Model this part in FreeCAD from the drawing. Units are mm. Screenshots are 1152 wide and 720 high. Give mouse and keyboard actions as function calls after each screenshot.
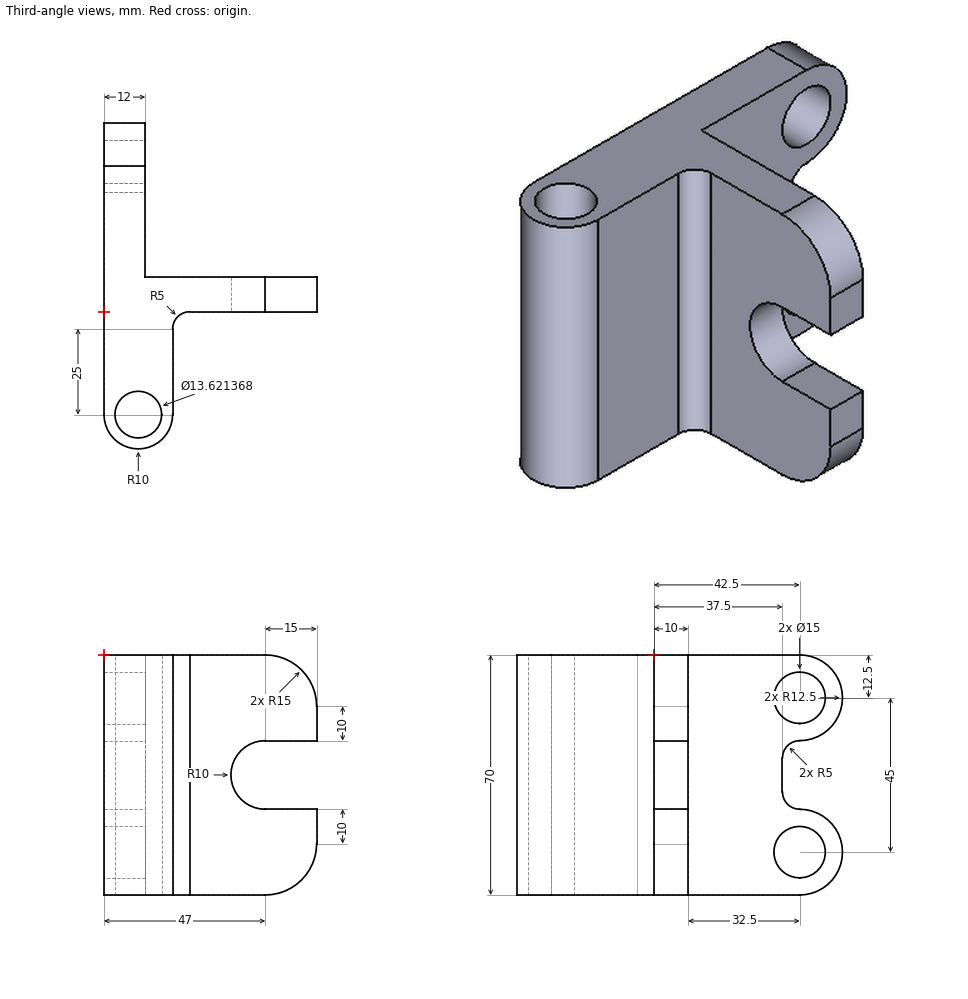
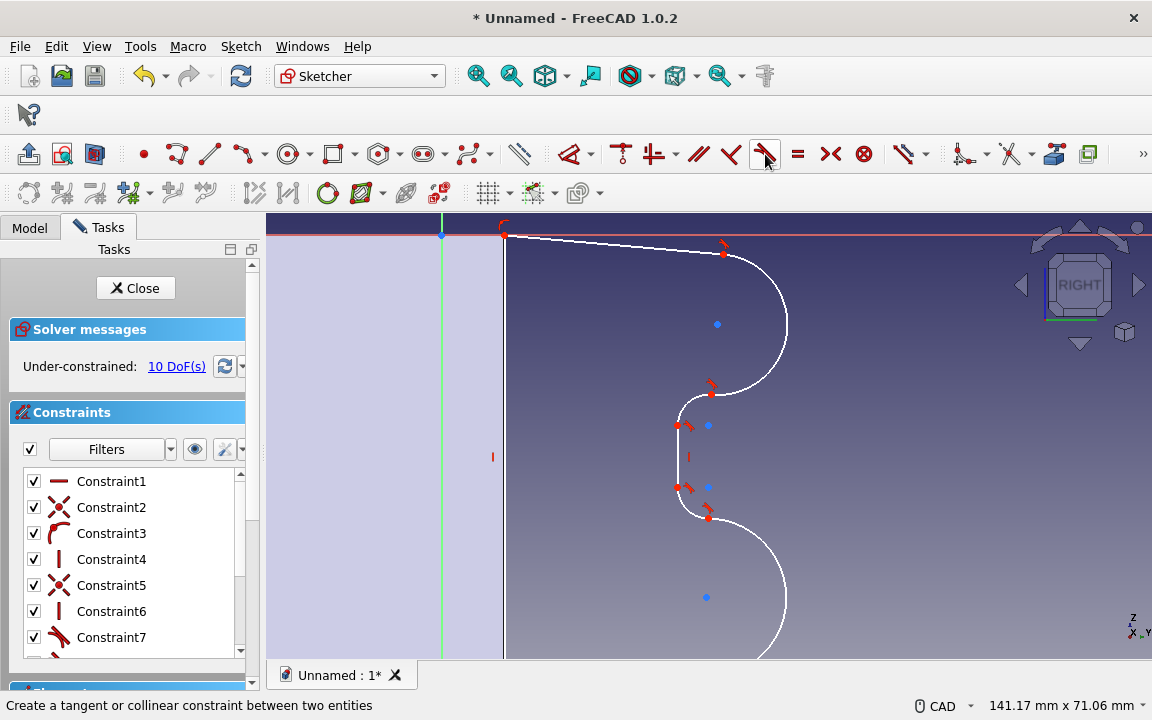
click(658, 249)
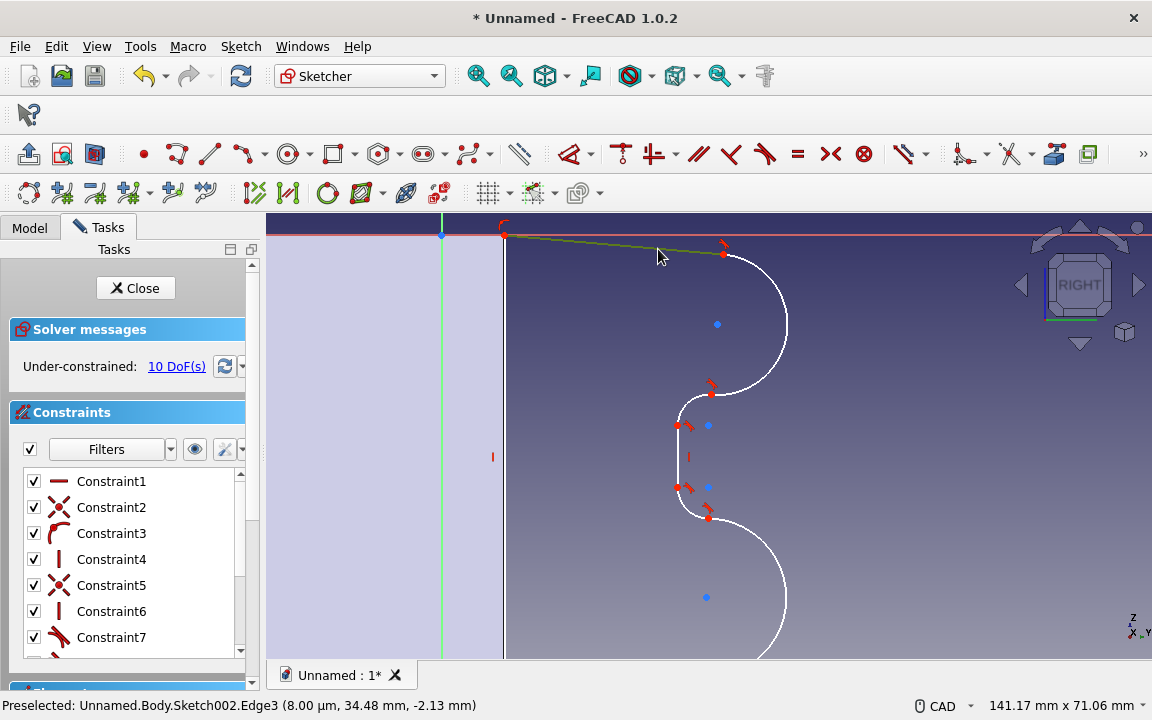
key(h)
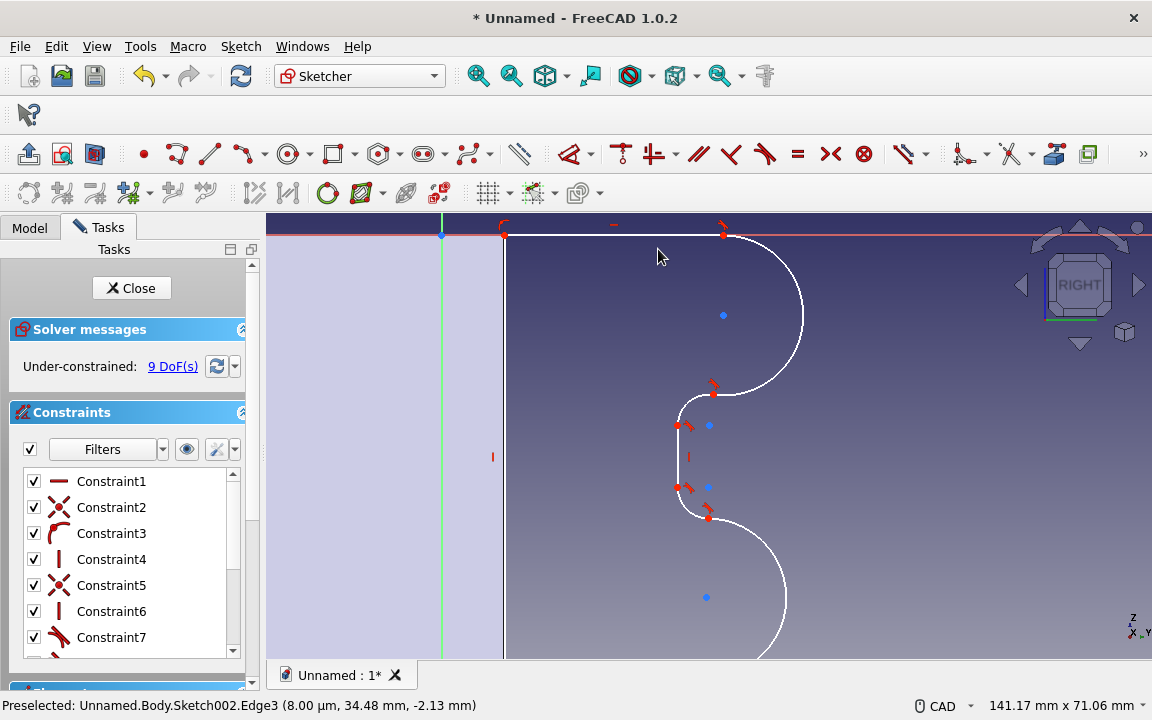
click(697, 397)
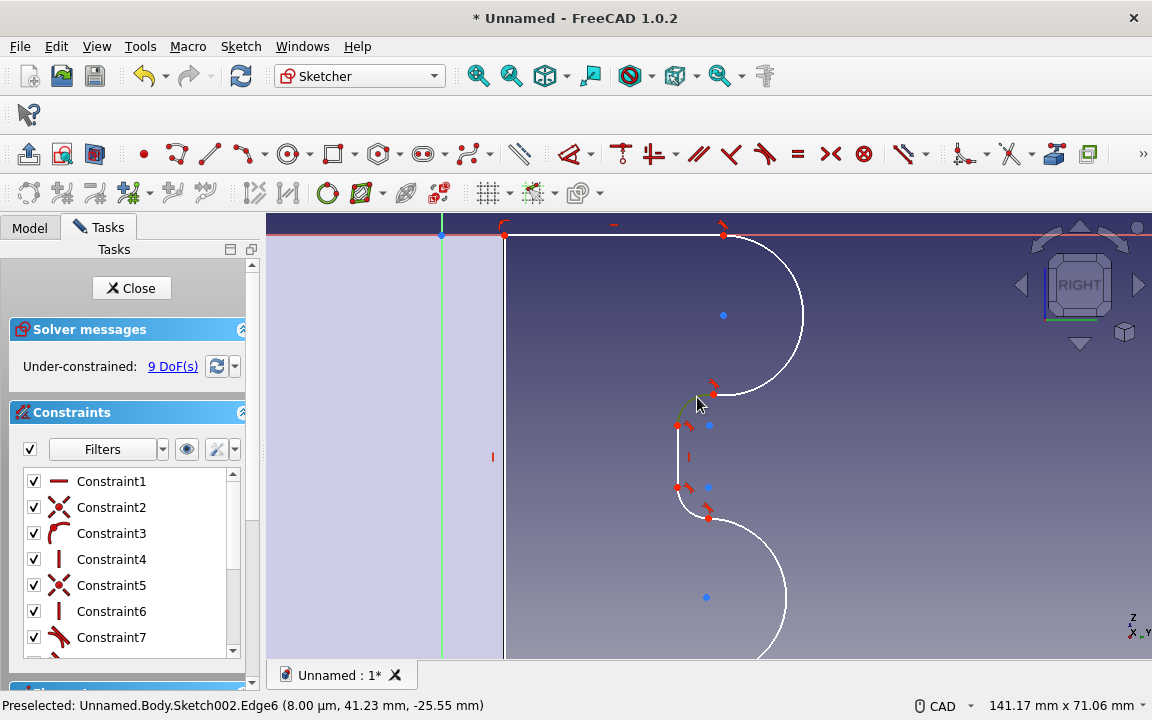
click(681, 502)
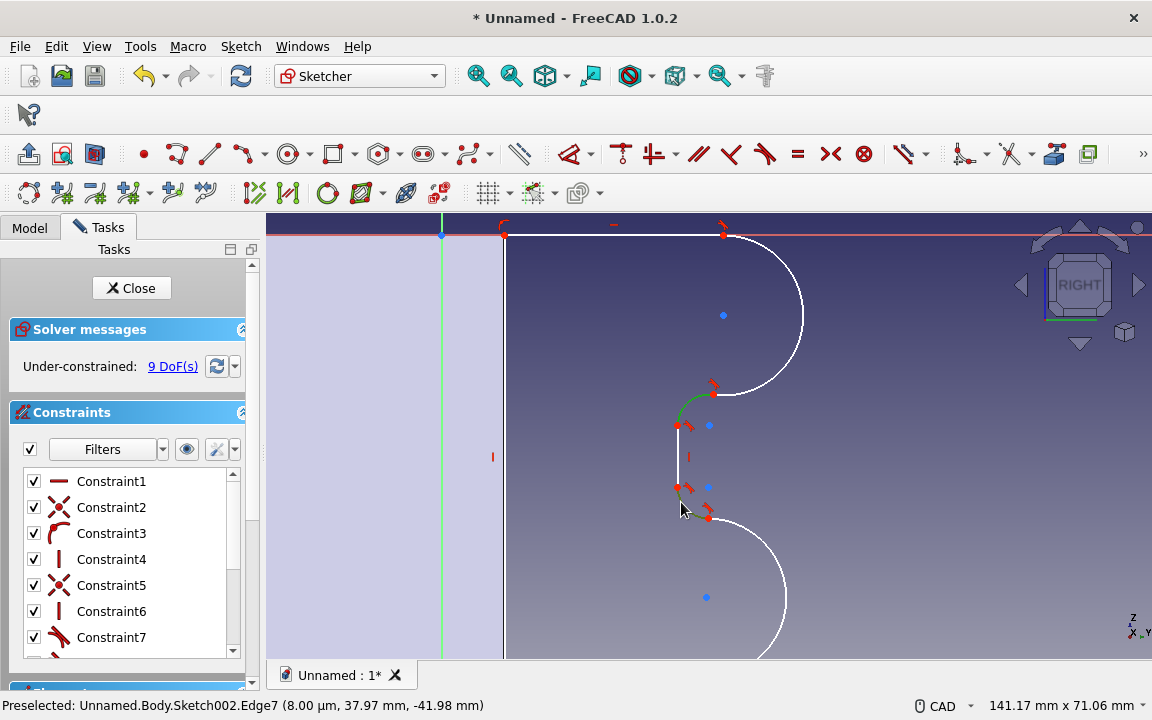
click(798, 154)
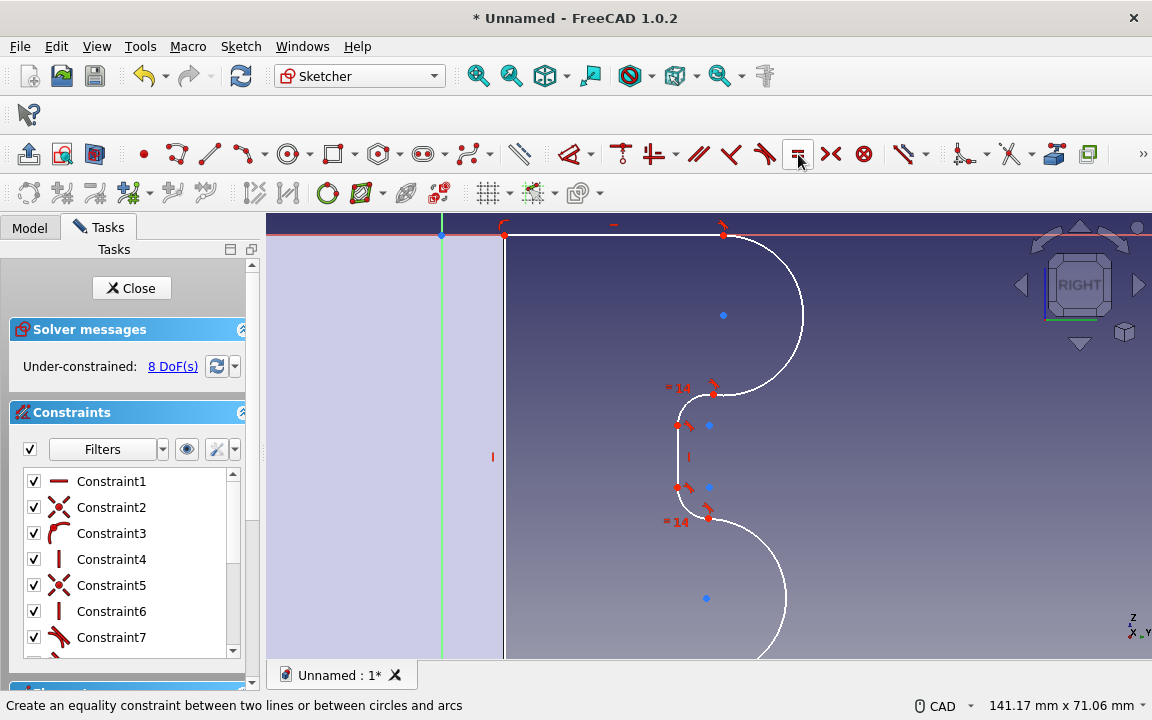
click(784, 368)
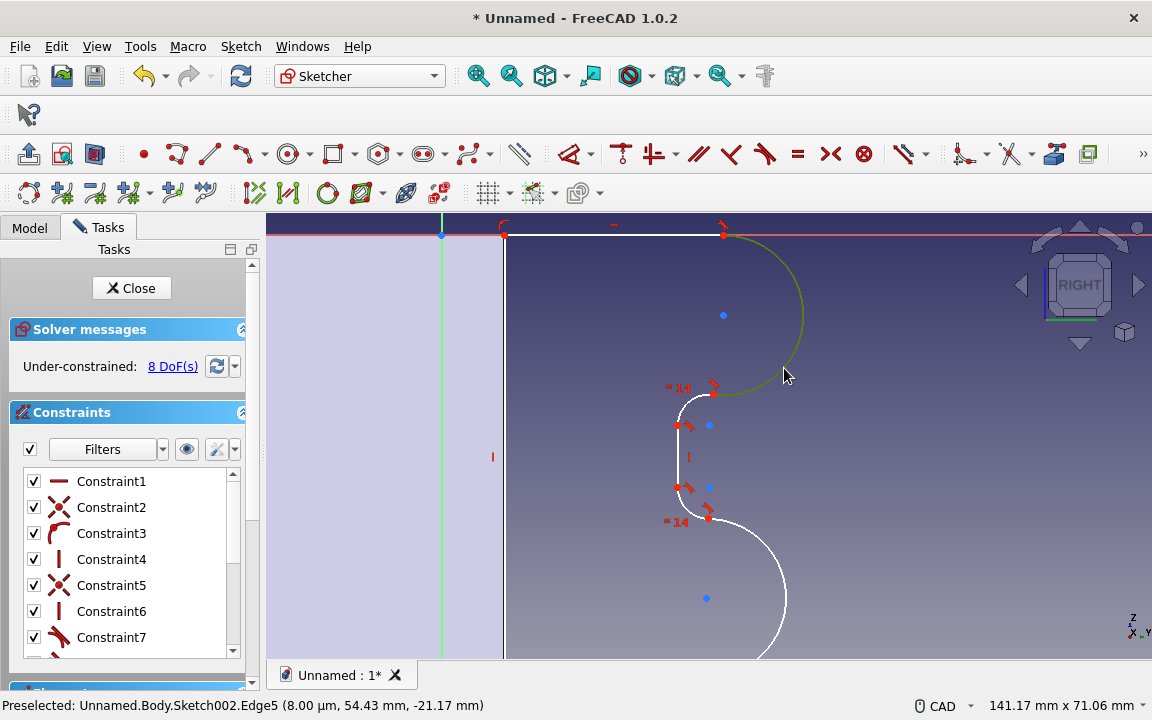
click(772, 552)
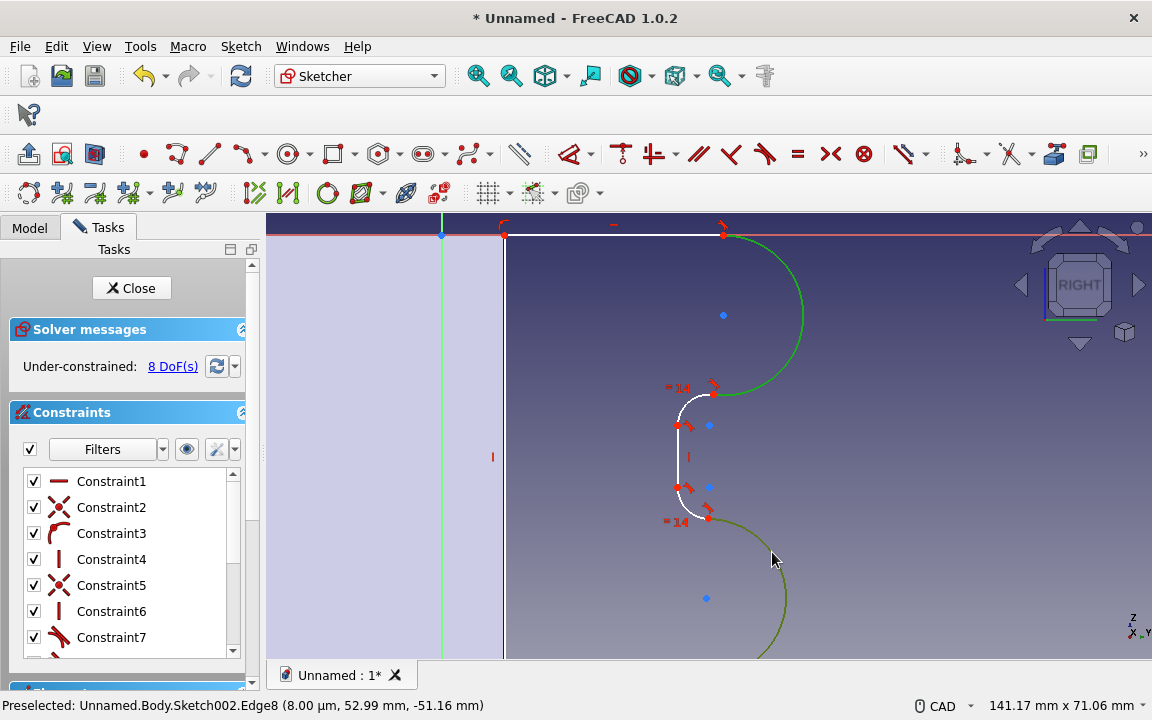
click(798, 154)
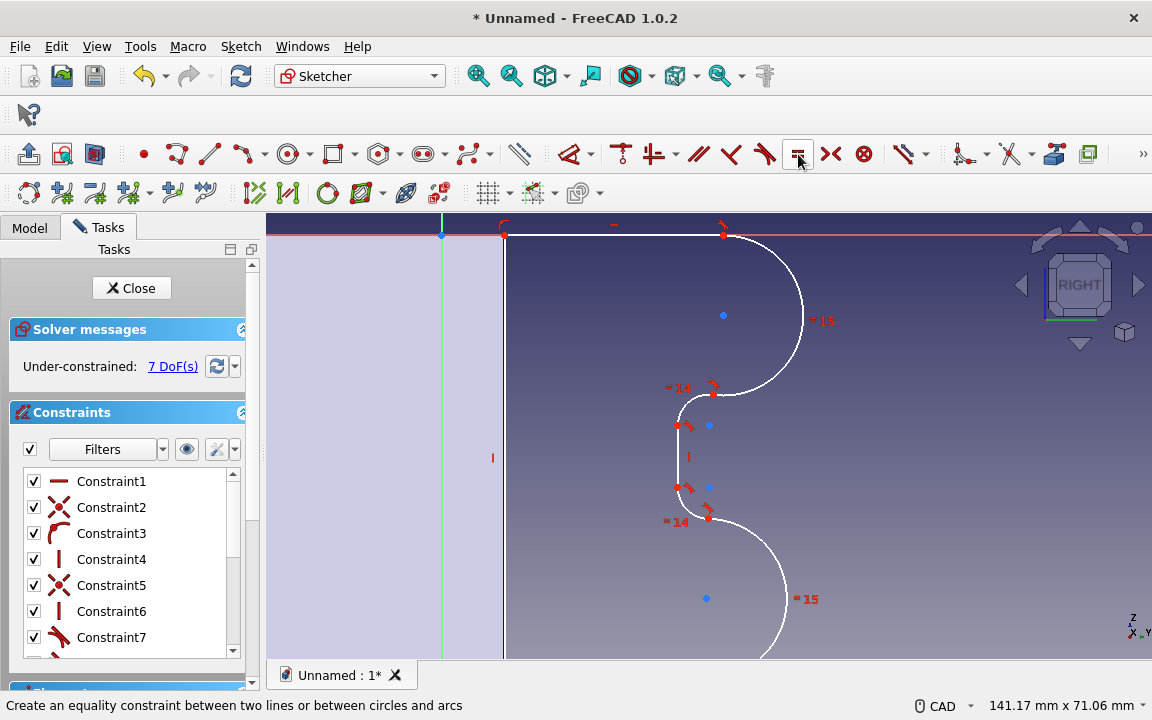
click(568, 154)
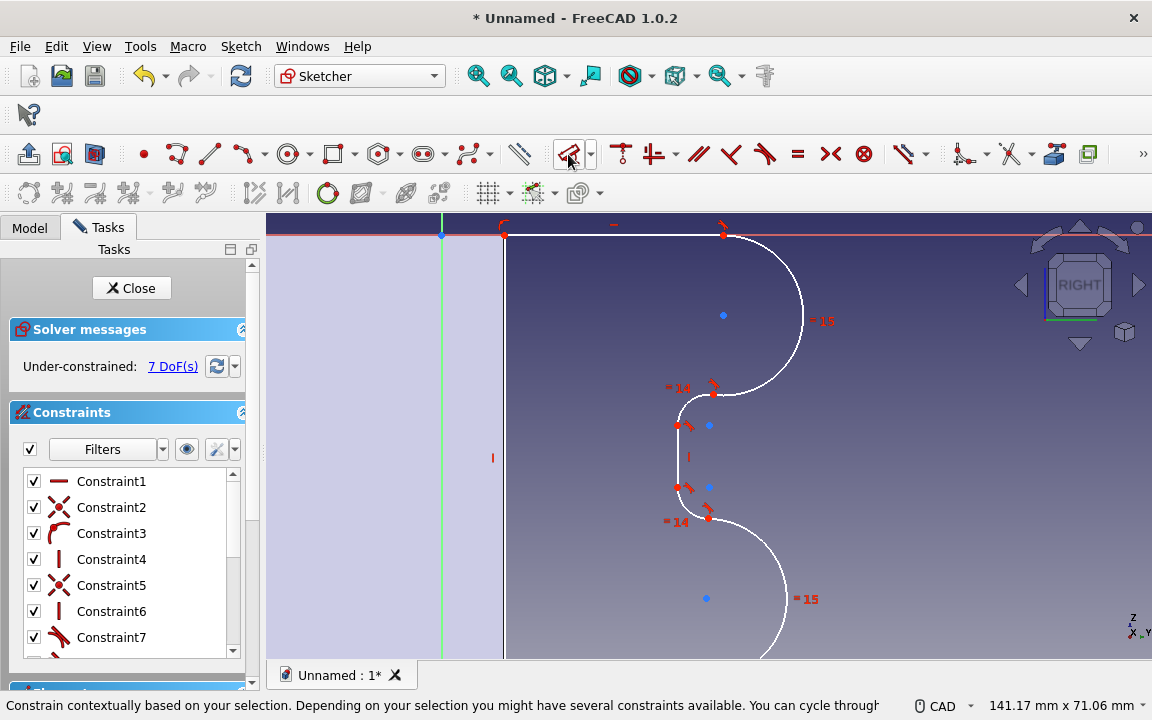
click(784, 368)
click(808, 389)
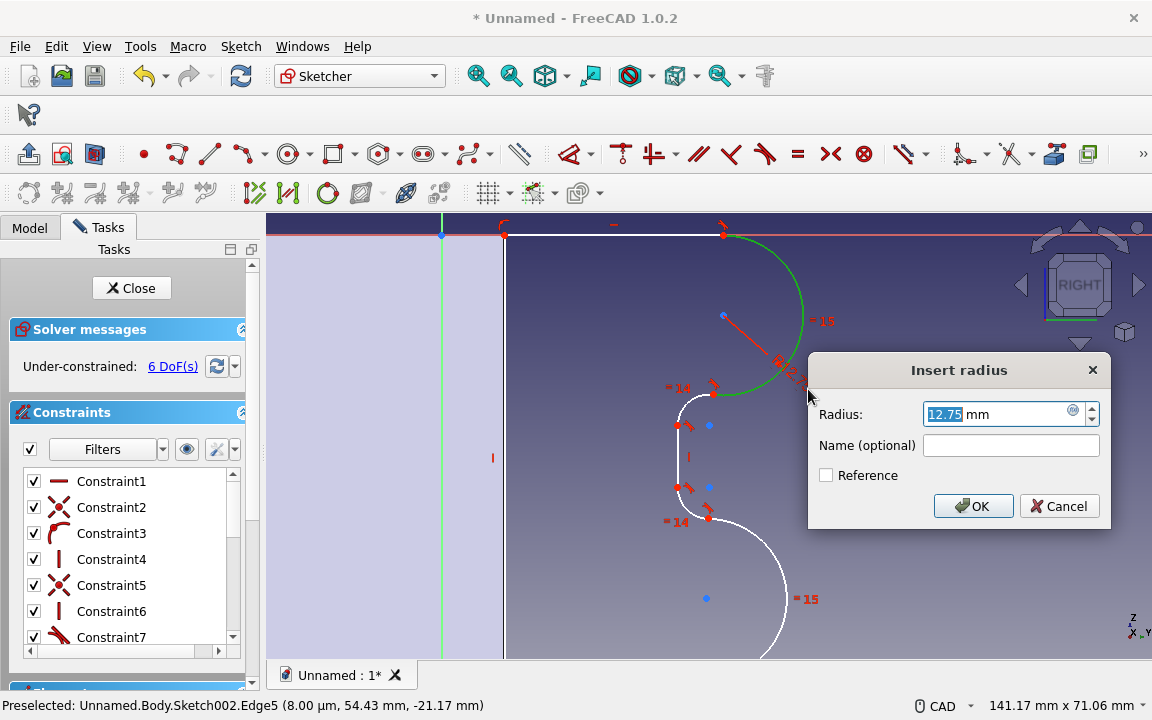
text(12.5)
key(Return)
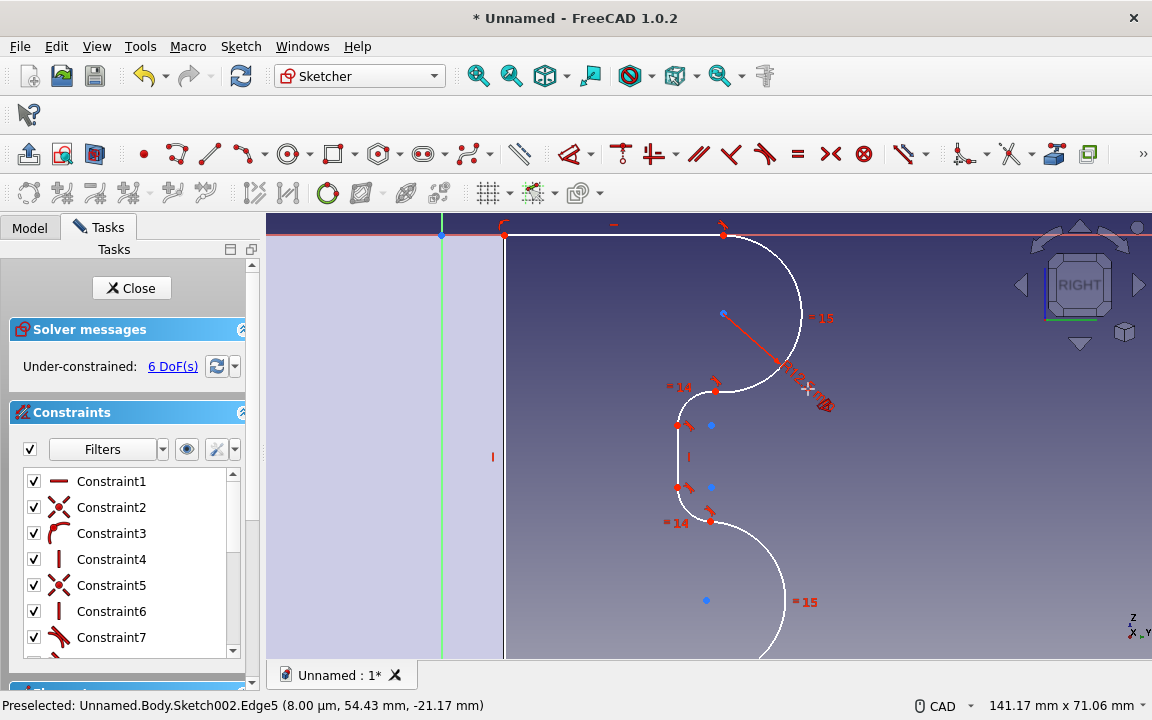
scroll(699, 394, up, 2)